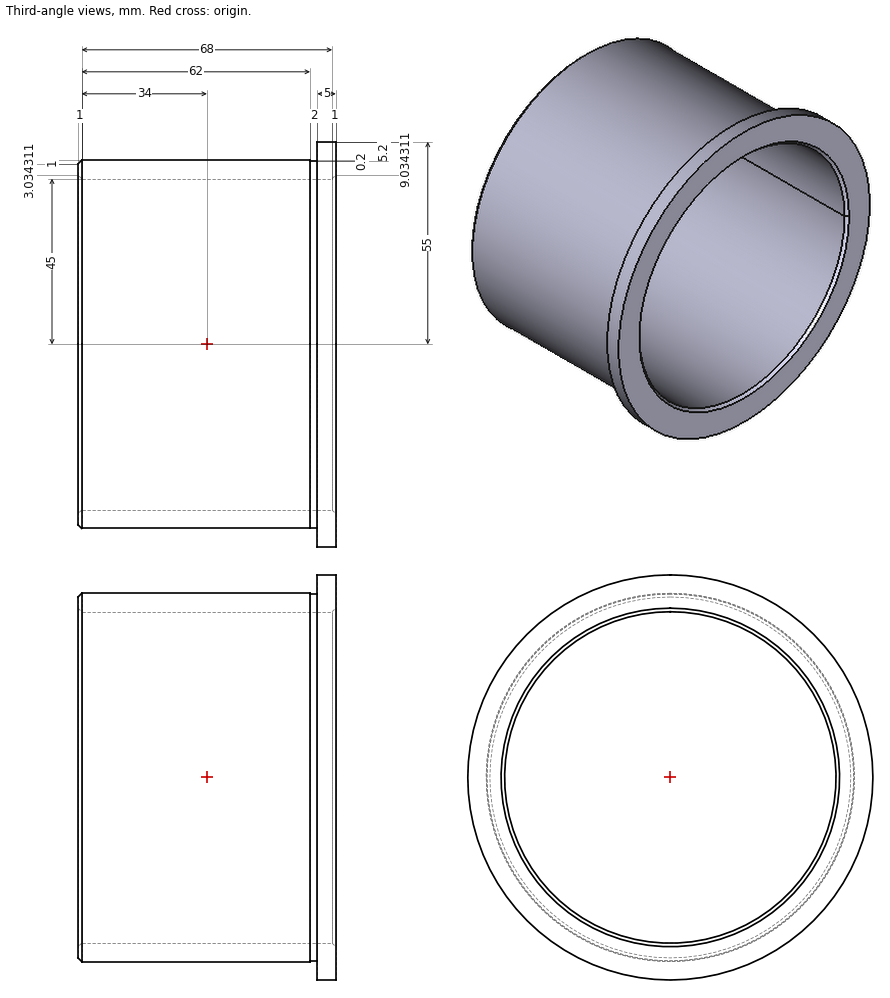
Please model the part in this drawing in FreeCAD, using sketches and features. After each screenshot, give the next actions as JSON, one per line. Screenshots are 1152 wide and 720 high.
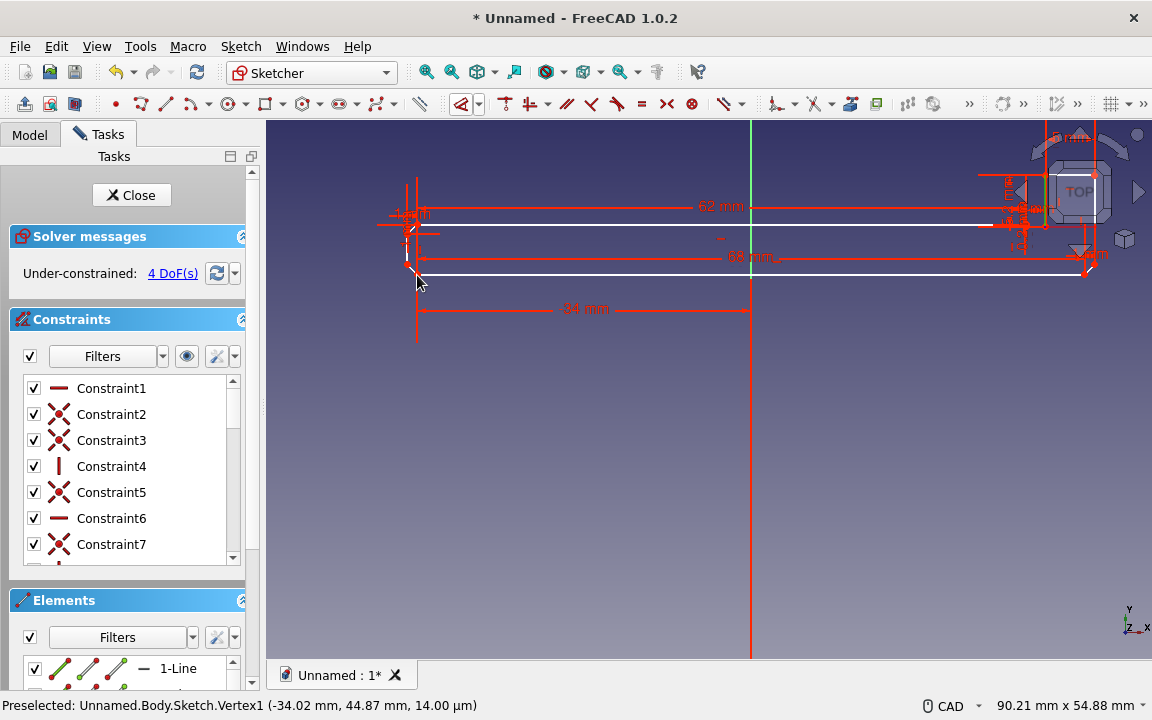
{"action": "left_click", "coordinate": [417, 275]}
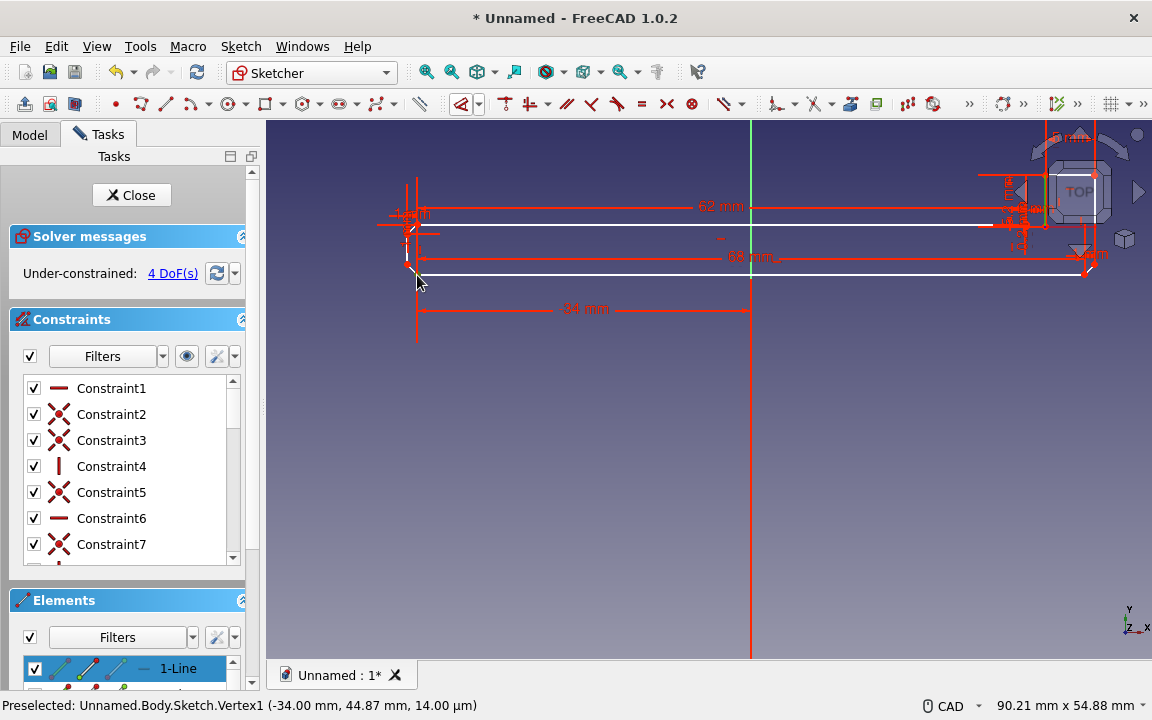
{"action": "key", "text": "i"}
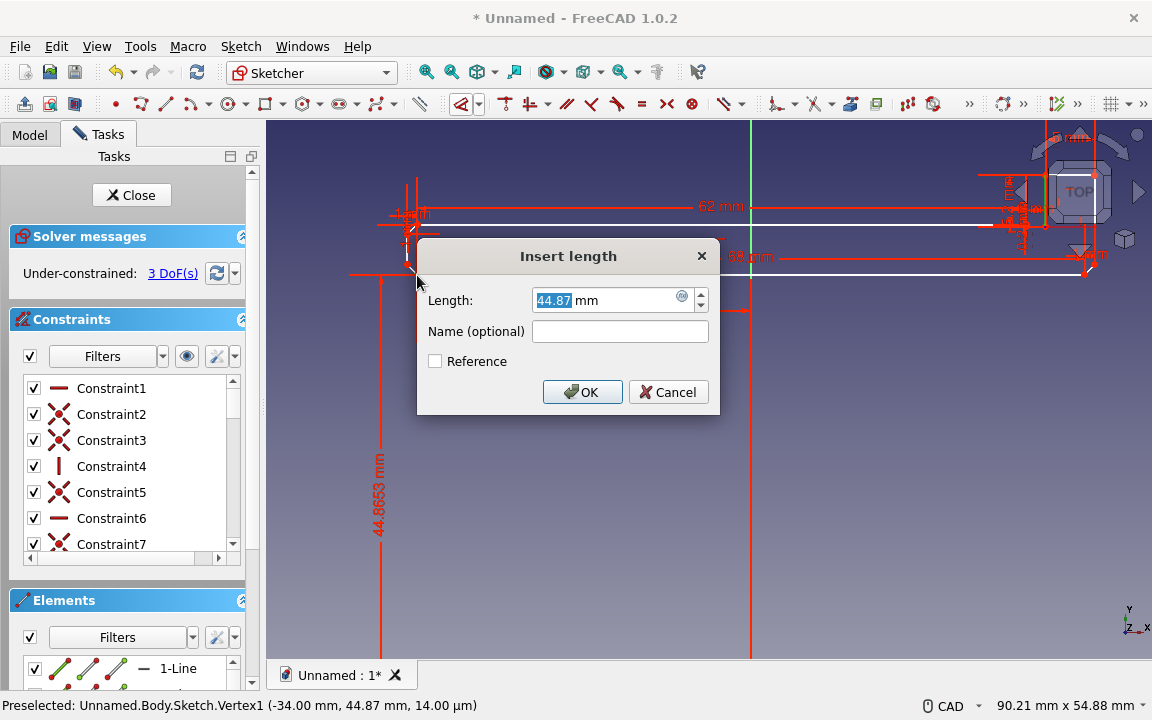
{"action": "type", "text": "45"}
{"action": "key", "text": "Return"}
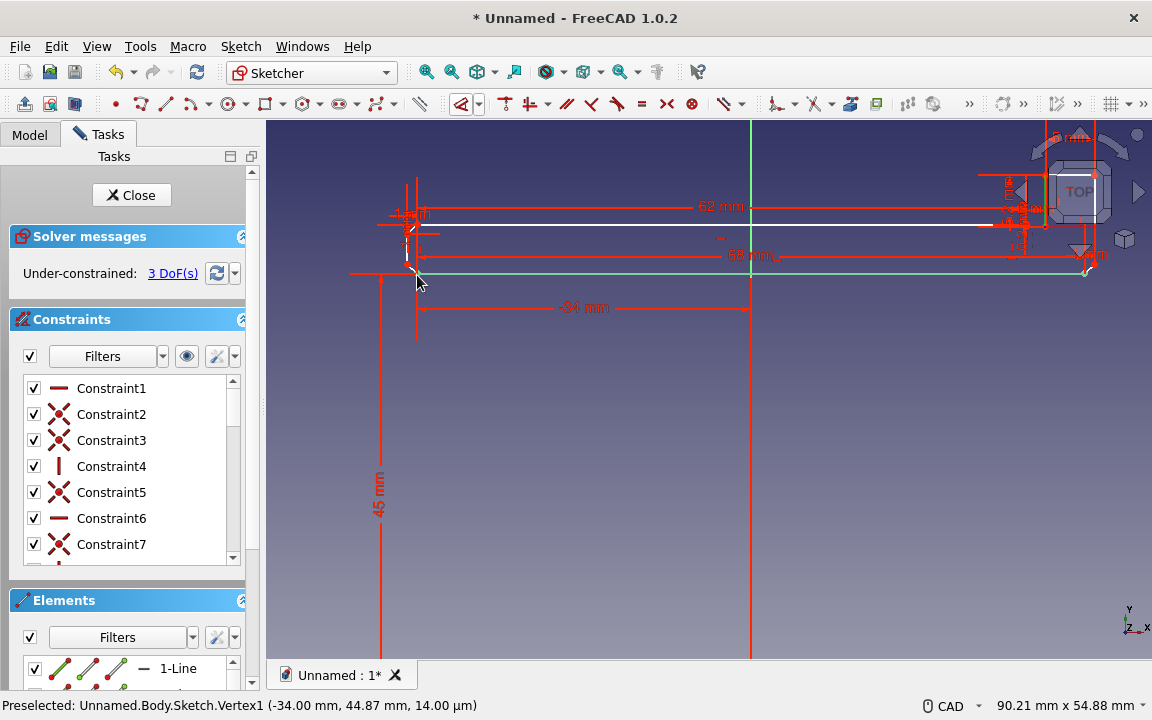
{"action": "scroll", "coordinate": [416, 276], "scroll_direction": "down", "scroll_amount": 2}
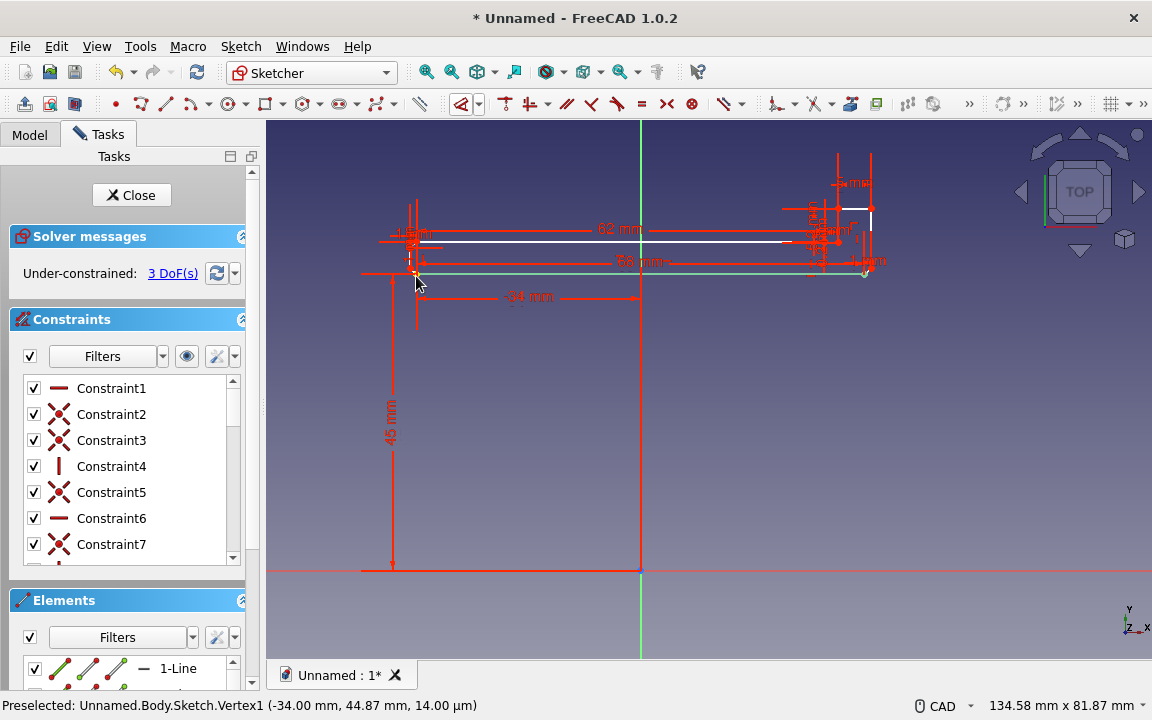
{"action": "left_click", "coordinate": [871, 209]}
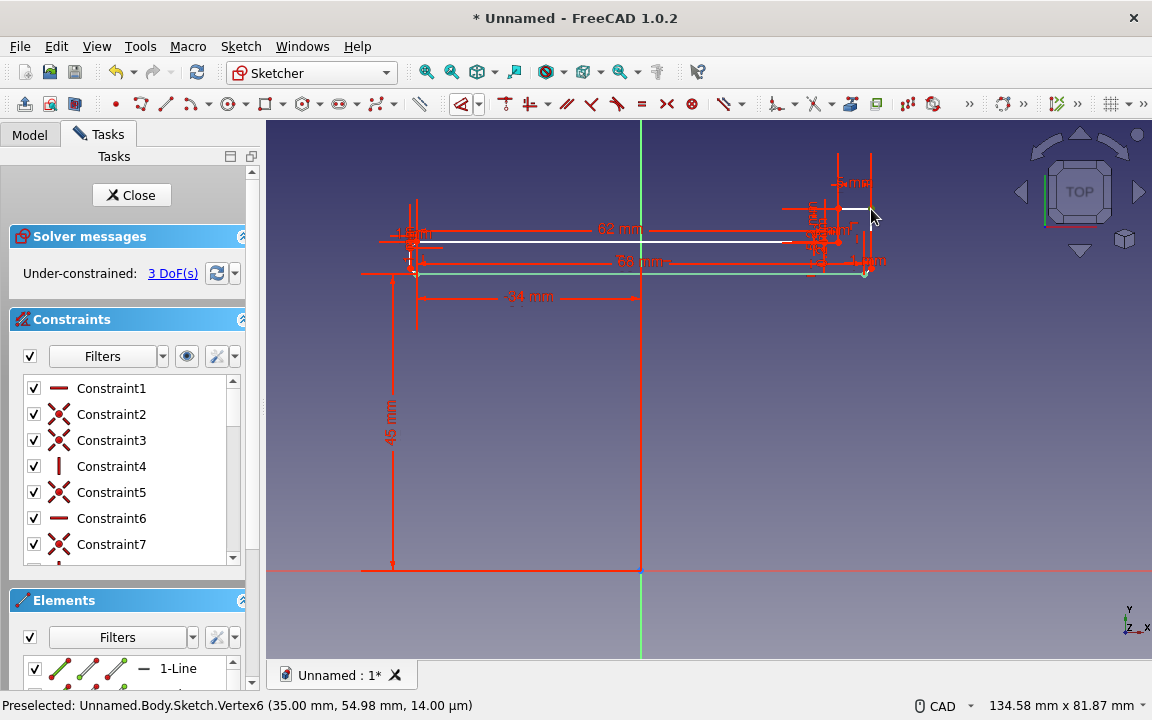
{"action": "left_click", "coordinate": [478, 104]}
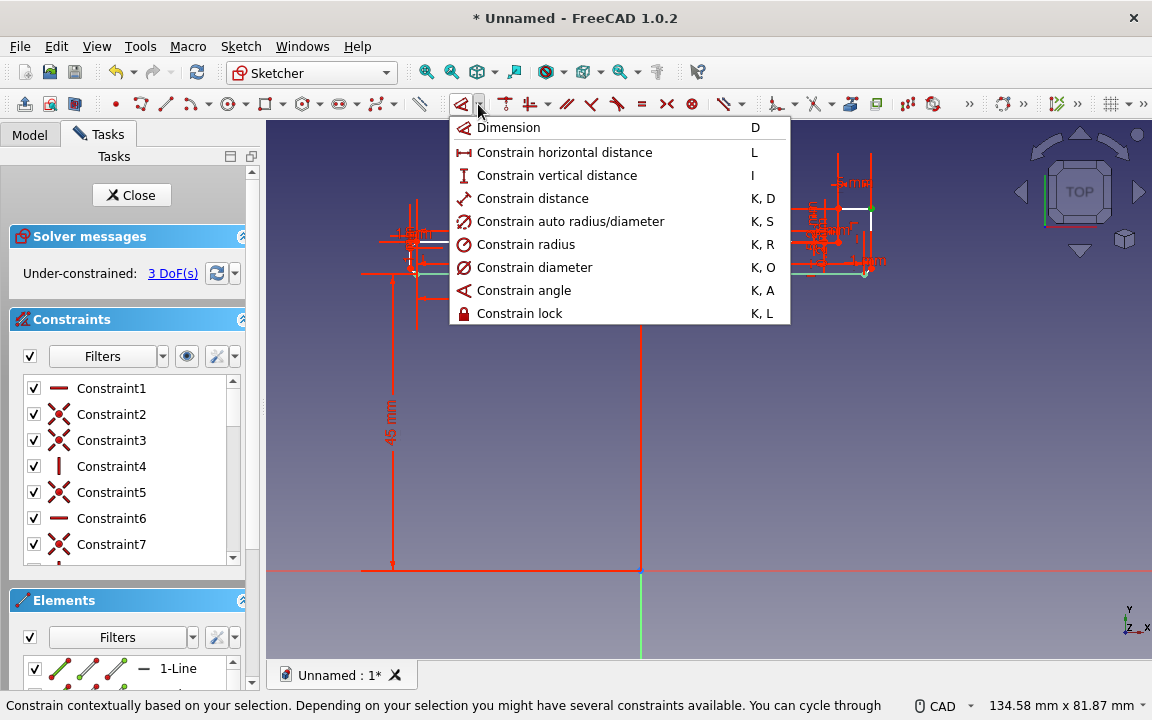
{"action": "left_click", "coordinate": [620, 176]}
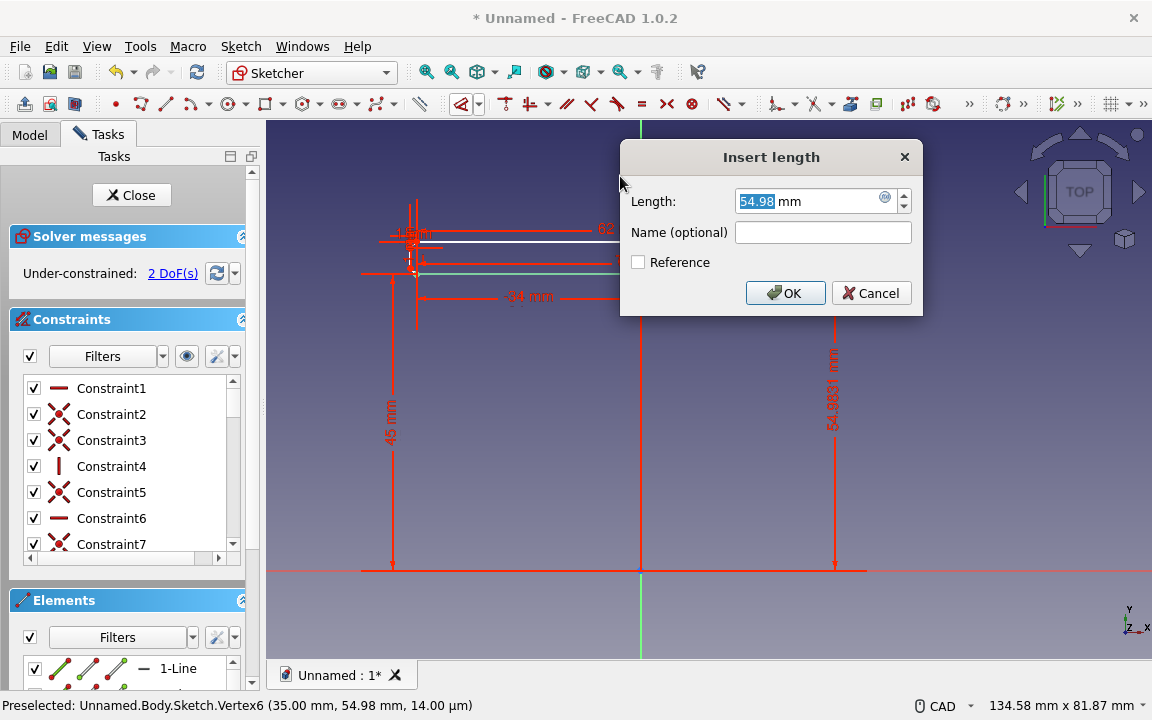
{"action": "type", "text": "55"}
{"action": "key", "text": "Return"}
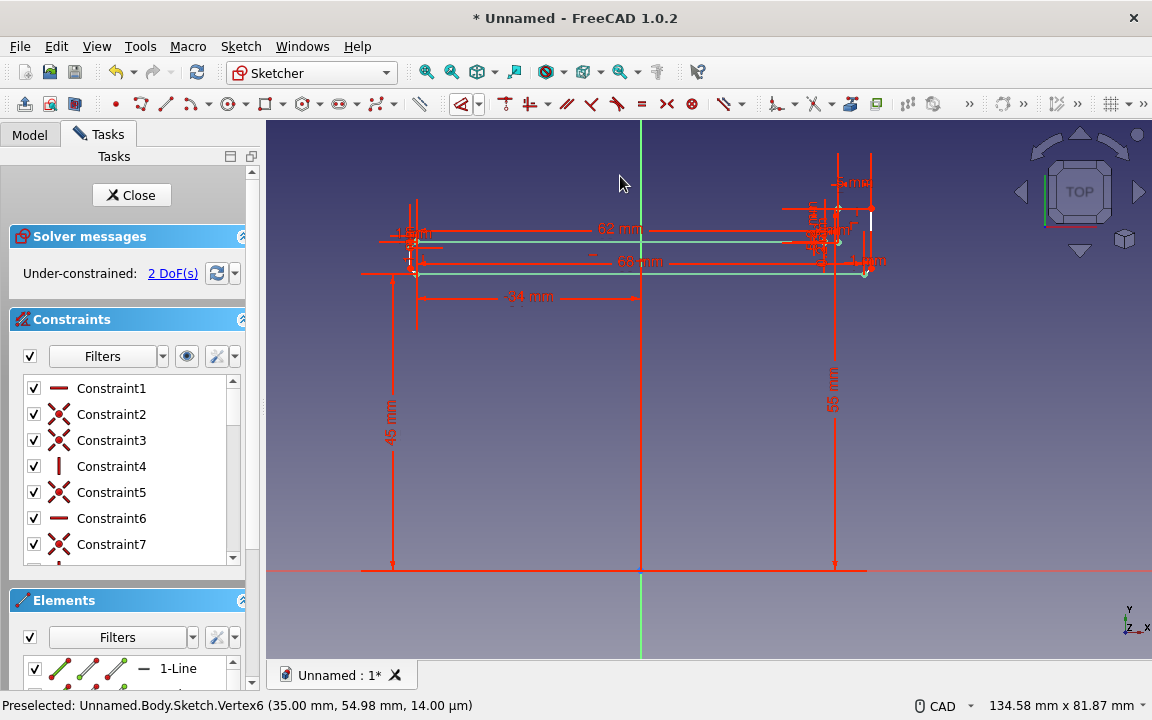
{"action": "left_click", "coordinate": [871, 250]}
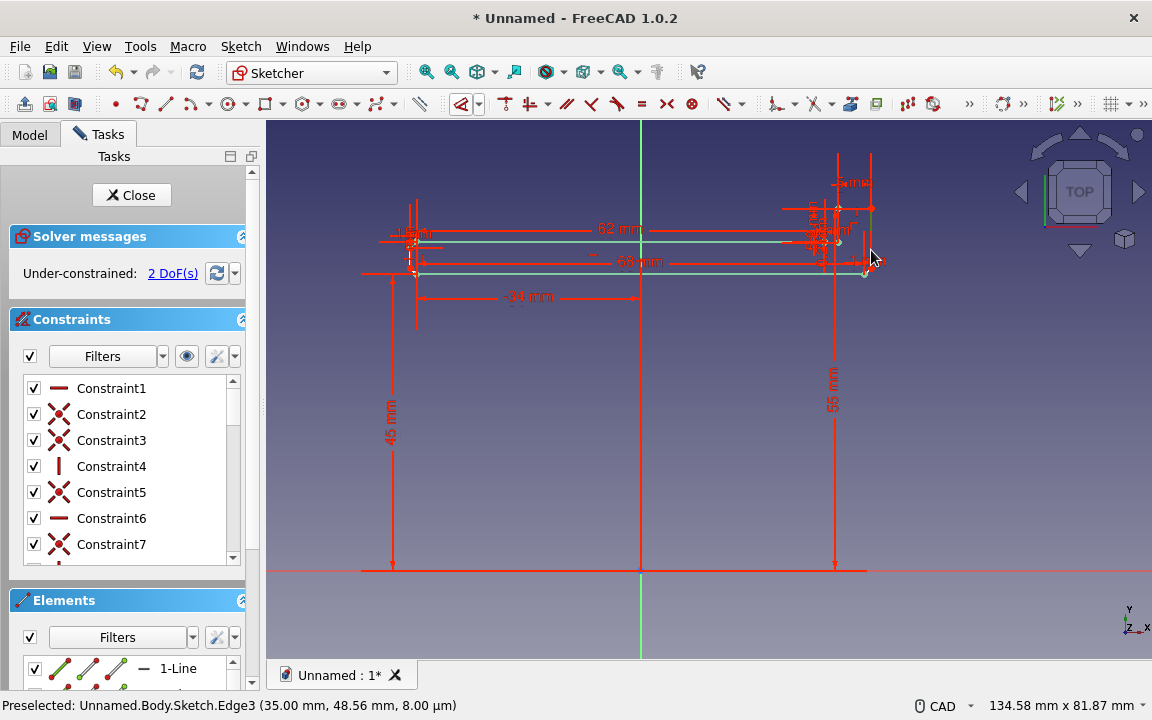
{"action": "key", "text": "i"}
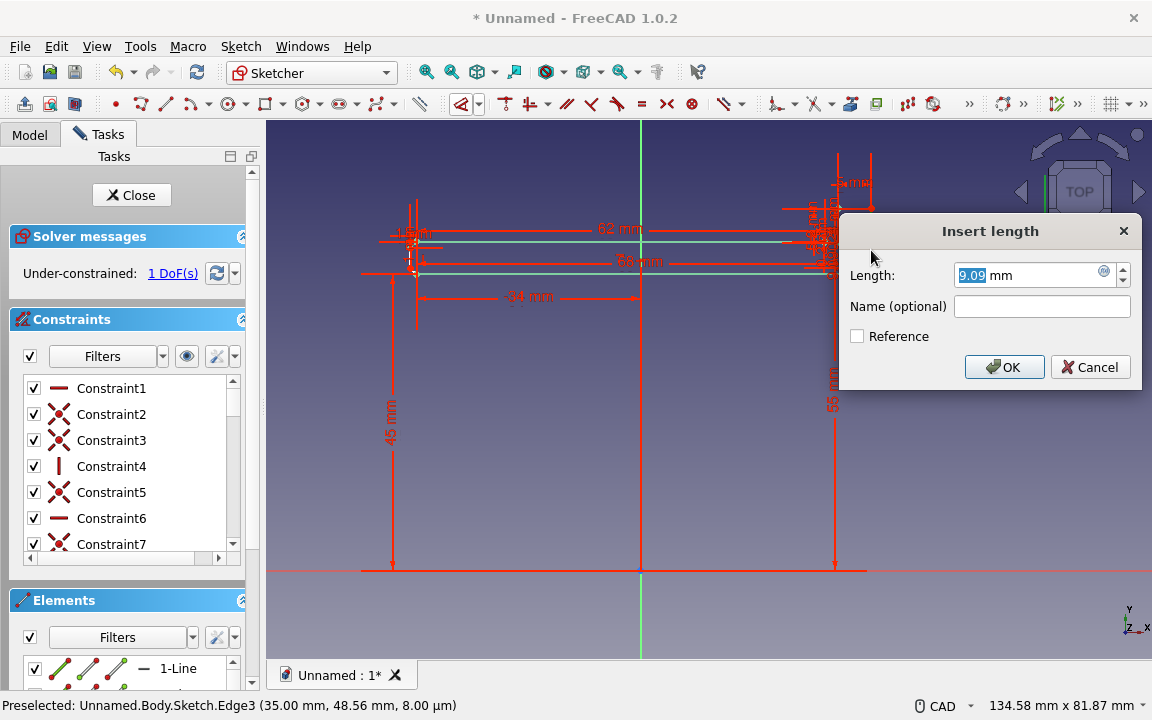
{"action": "type", "text": "9.034311"}
{"action": "key", "text": "Return"}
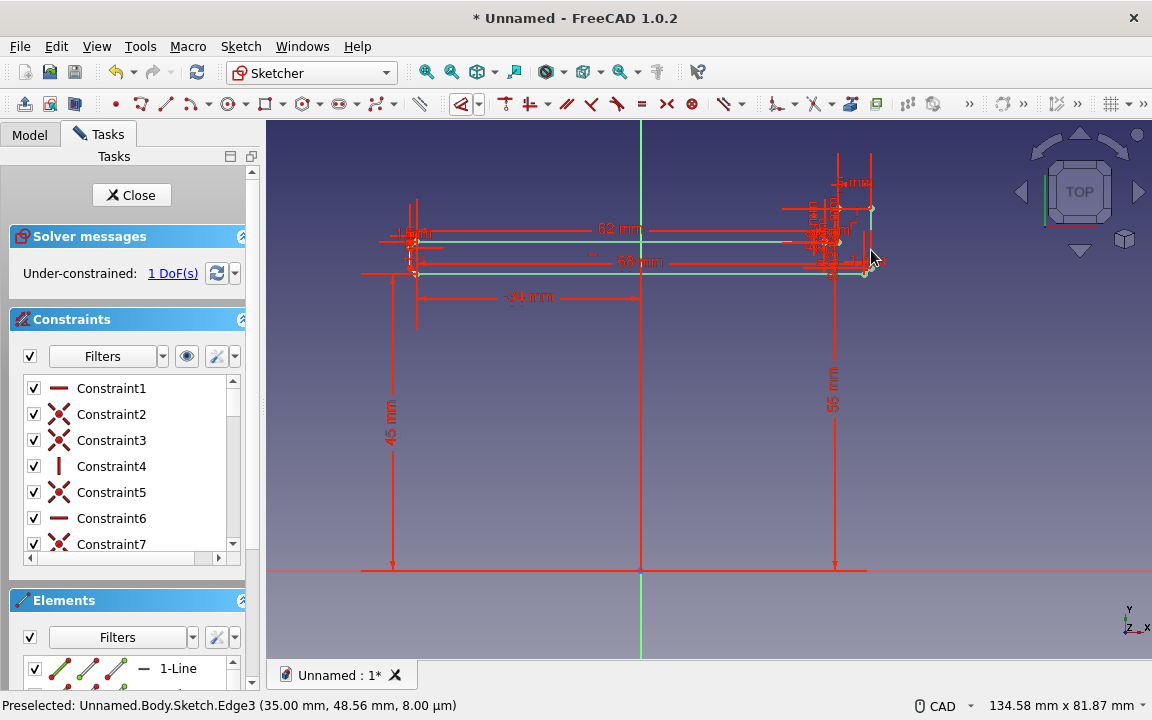
{"action": "scroll", "coordinate": [410, 258], "scroll_direction": "up", "scroll_amount": 4}